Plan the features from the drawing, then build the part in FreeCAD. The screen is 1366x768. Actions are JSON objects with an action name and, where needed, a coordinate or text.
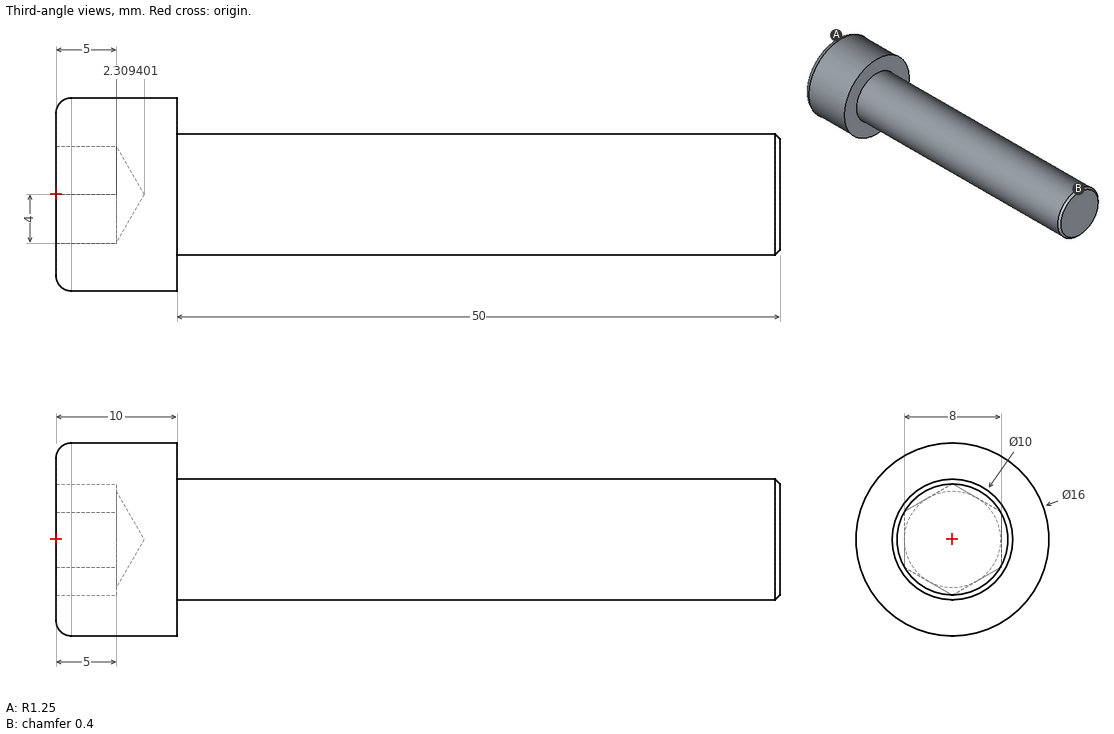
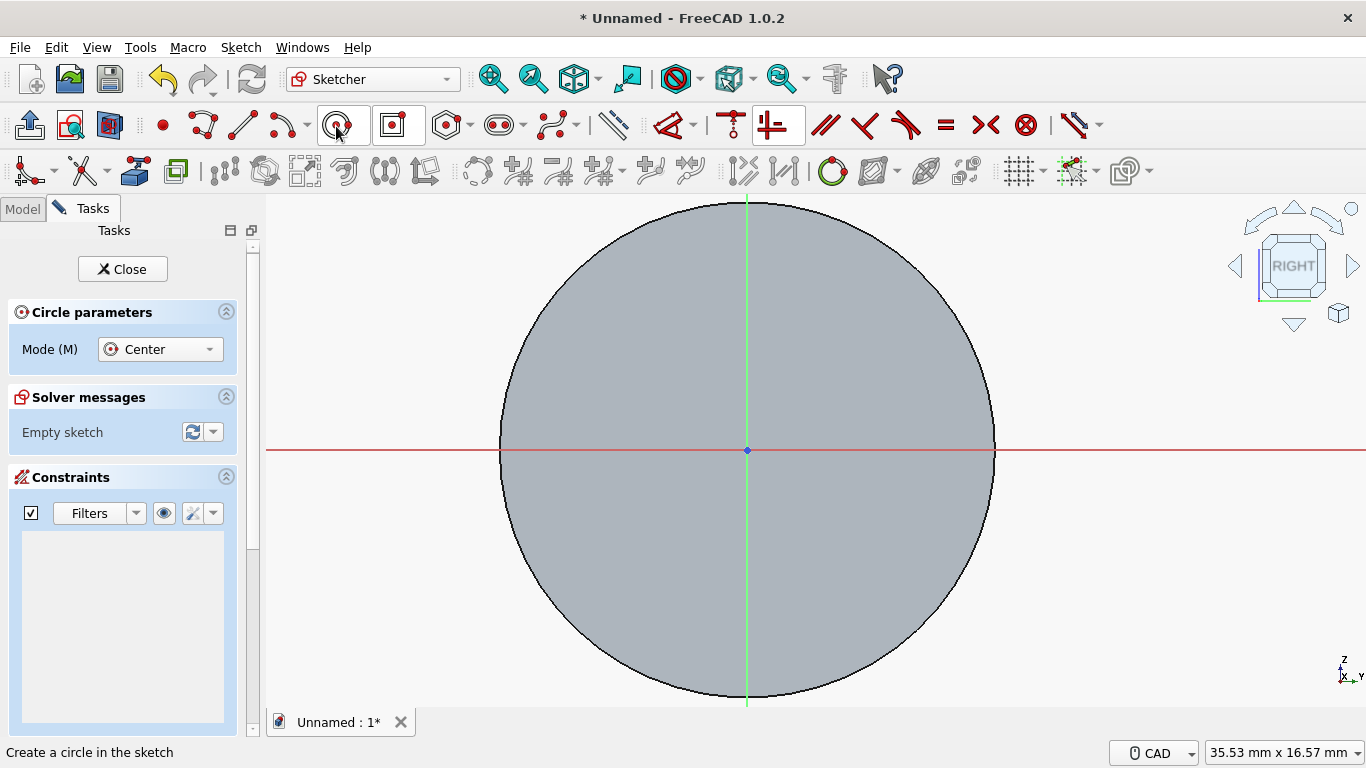
{"action": "left_click", "coordinate": [747, 450]}
{"action": "left_click", "coordinate": [857, 341]}
{"action": "key", "text": "Escape"}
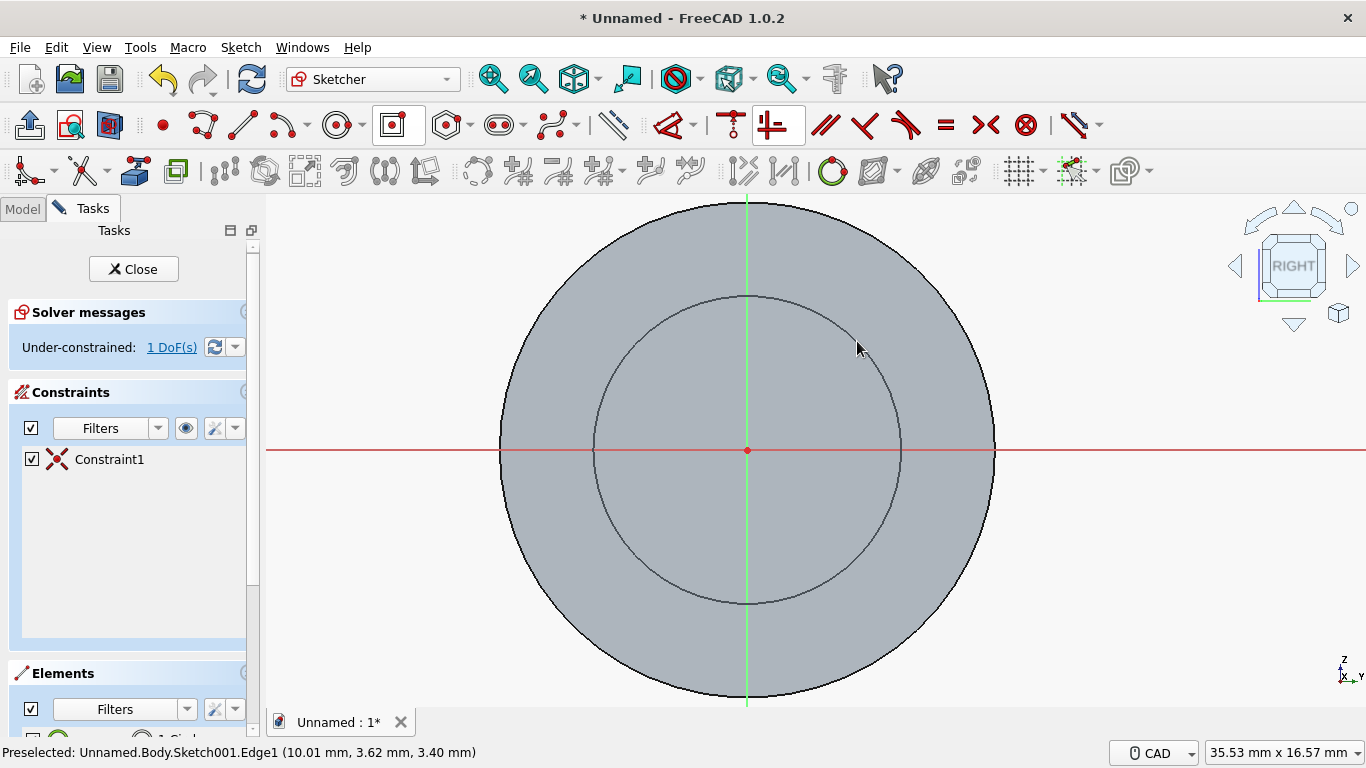
{"action": "left_click", "coordinate": [668, 126]}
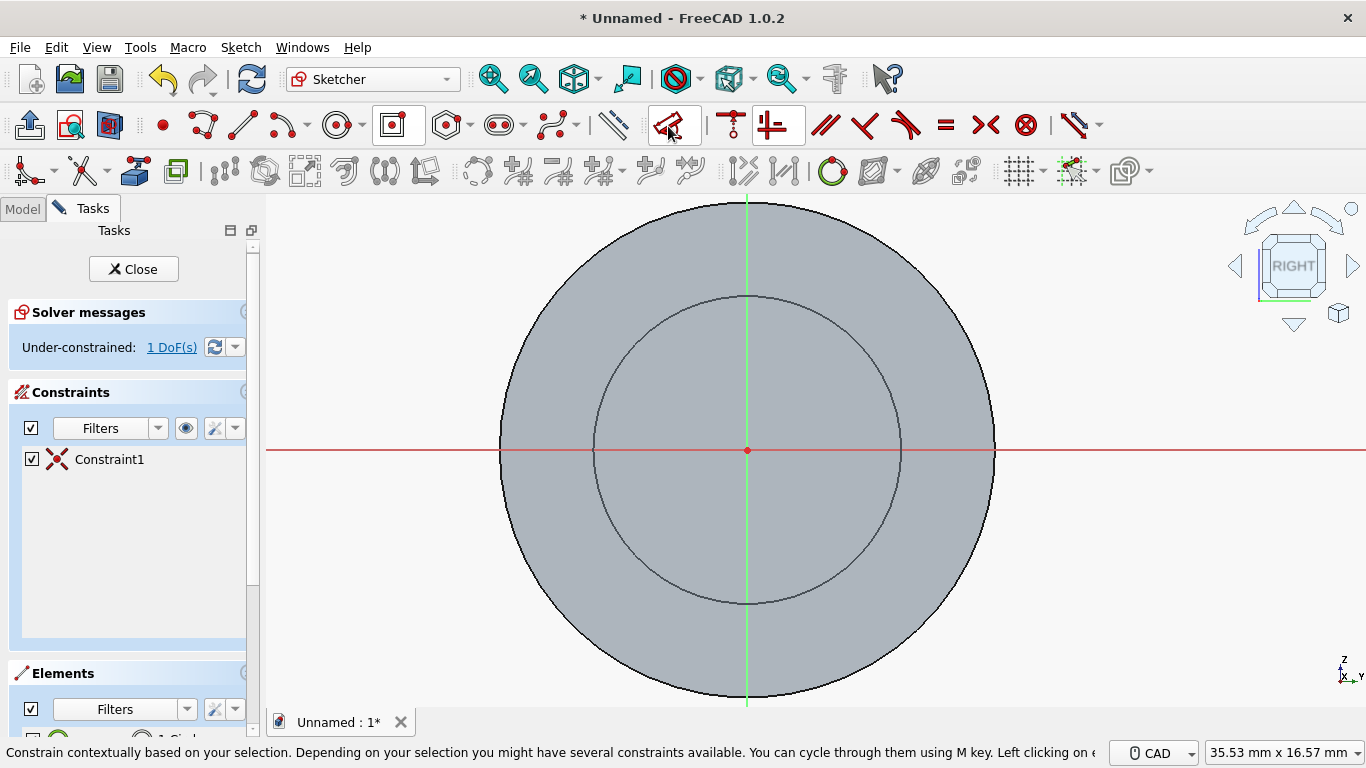
{"action": "left_click", "coordinate": [856, 341]}
{"action": "left_click", "coordinate": [879, 318]}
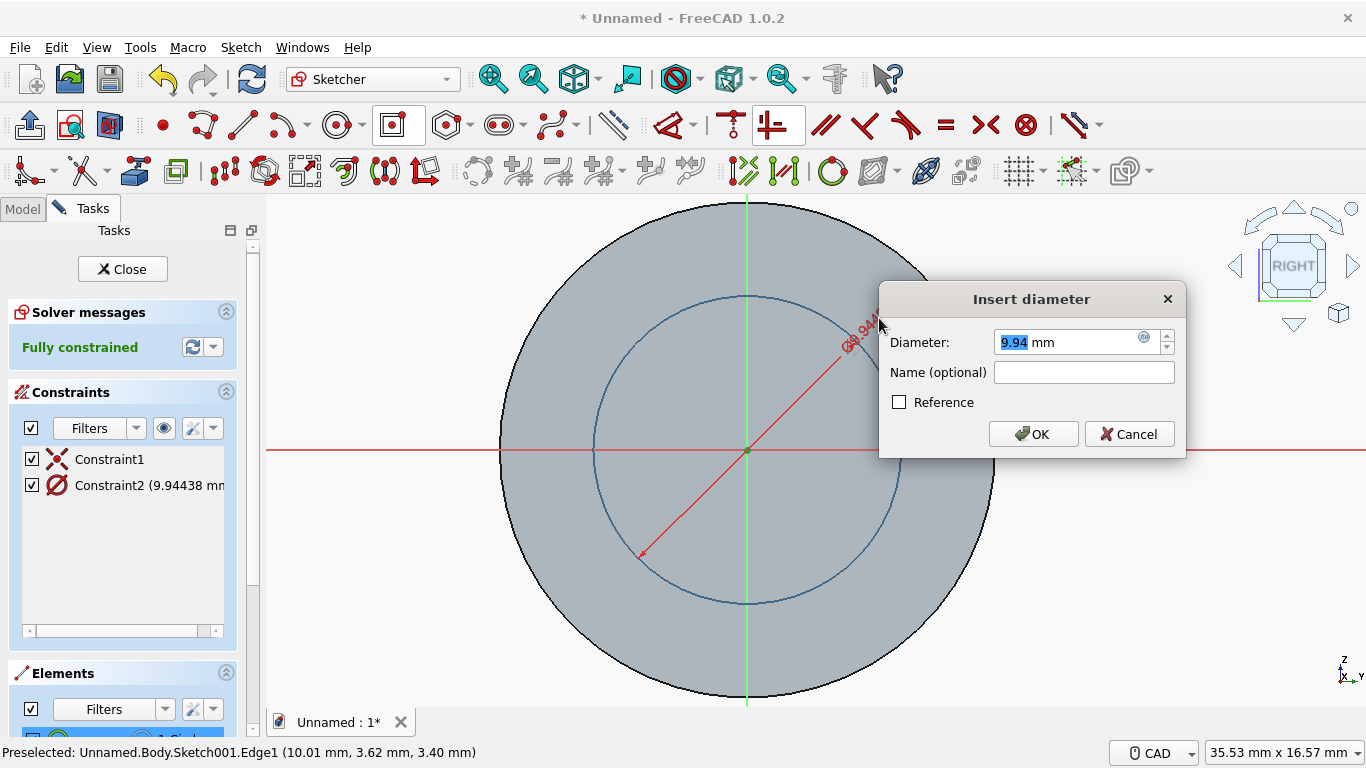
{"action": "type", "text": "10"}
{"action": "key", "text": "Return"}
{"action": "key", "text": "Escape"}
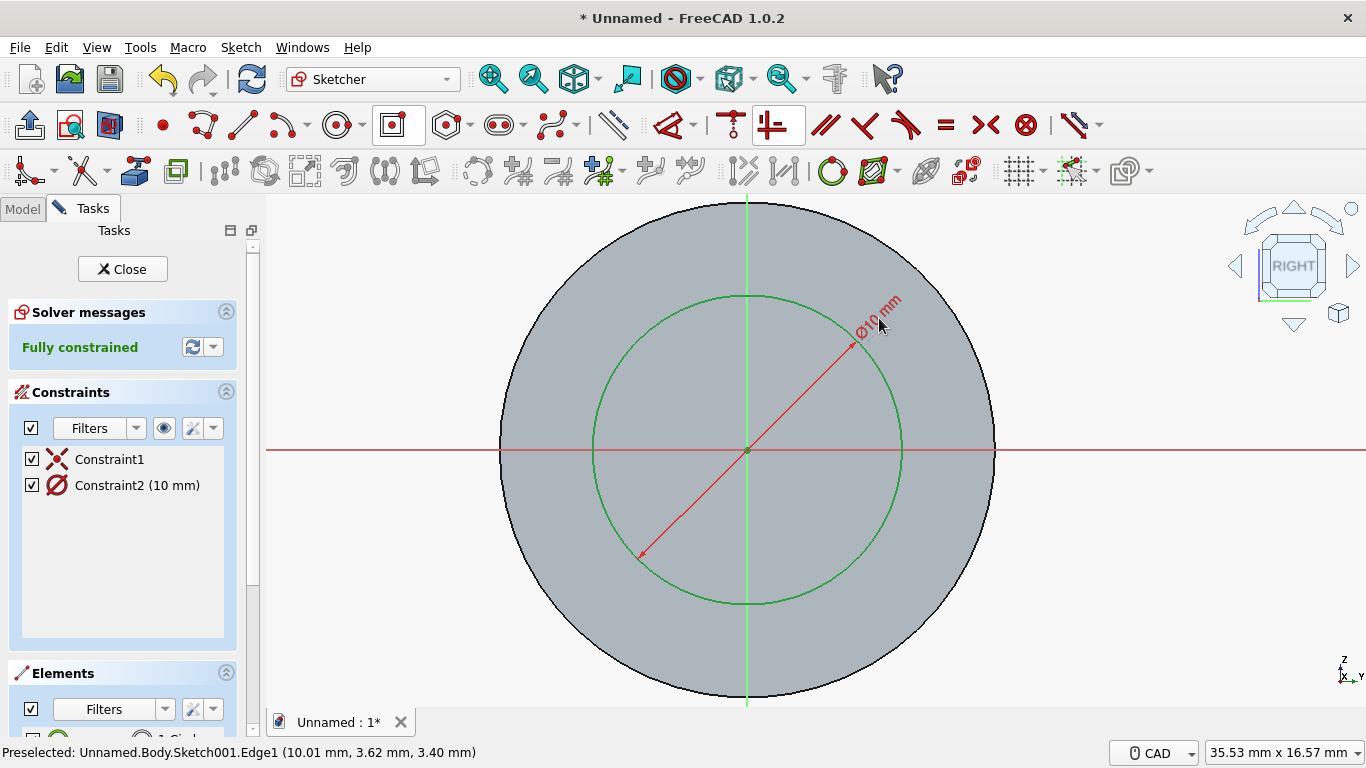
{"action": "left_click", "coordinate": [123, 269]}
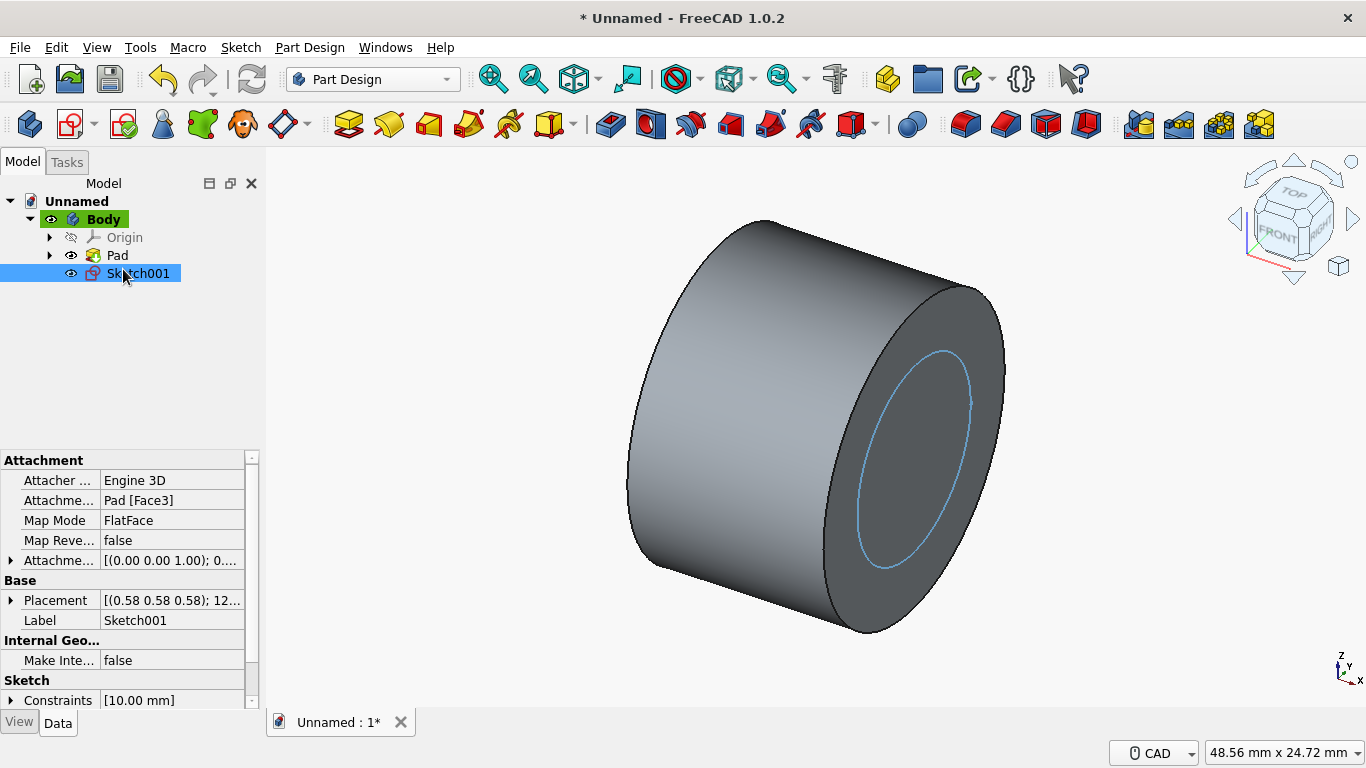
{"action": "left_click", "coordinate": [350, 124]}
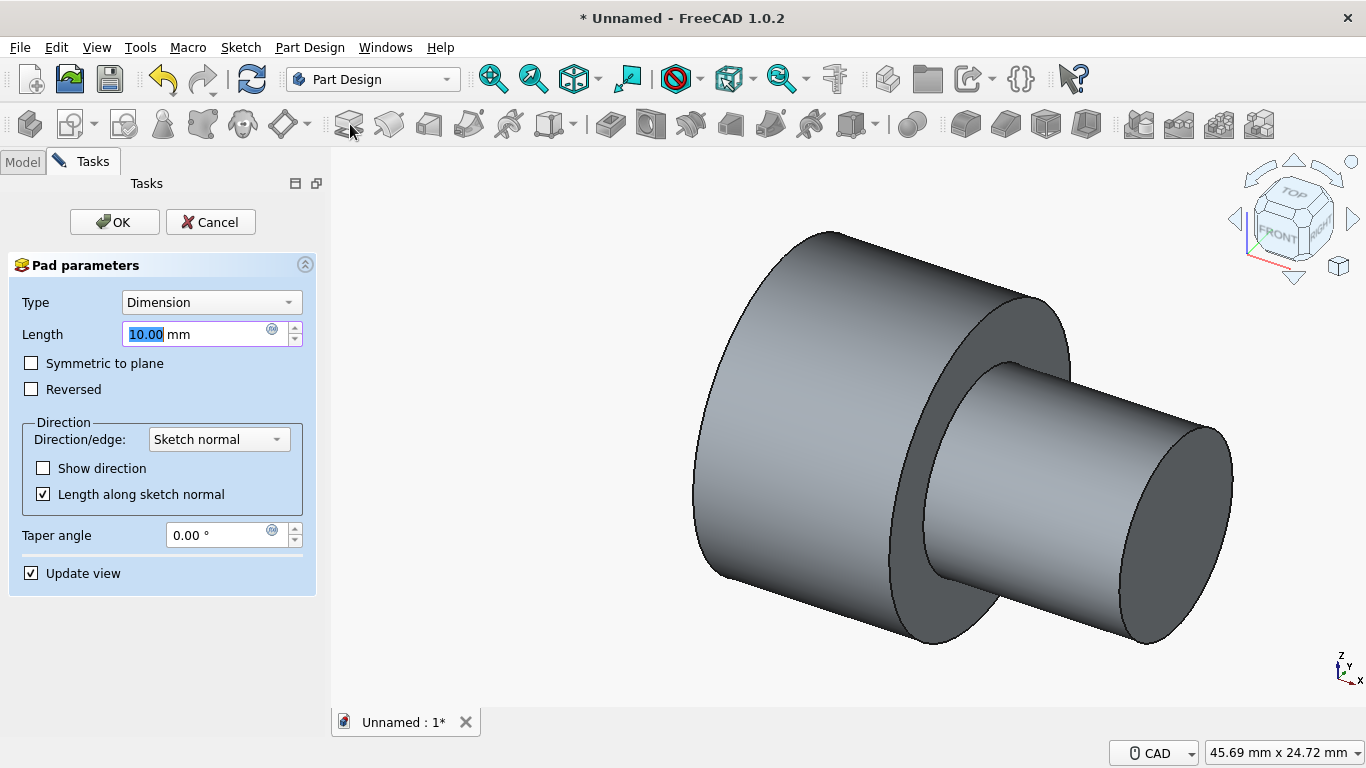
{"action": "type", "text": "50"}
{"action": "key", "text": "Tab"}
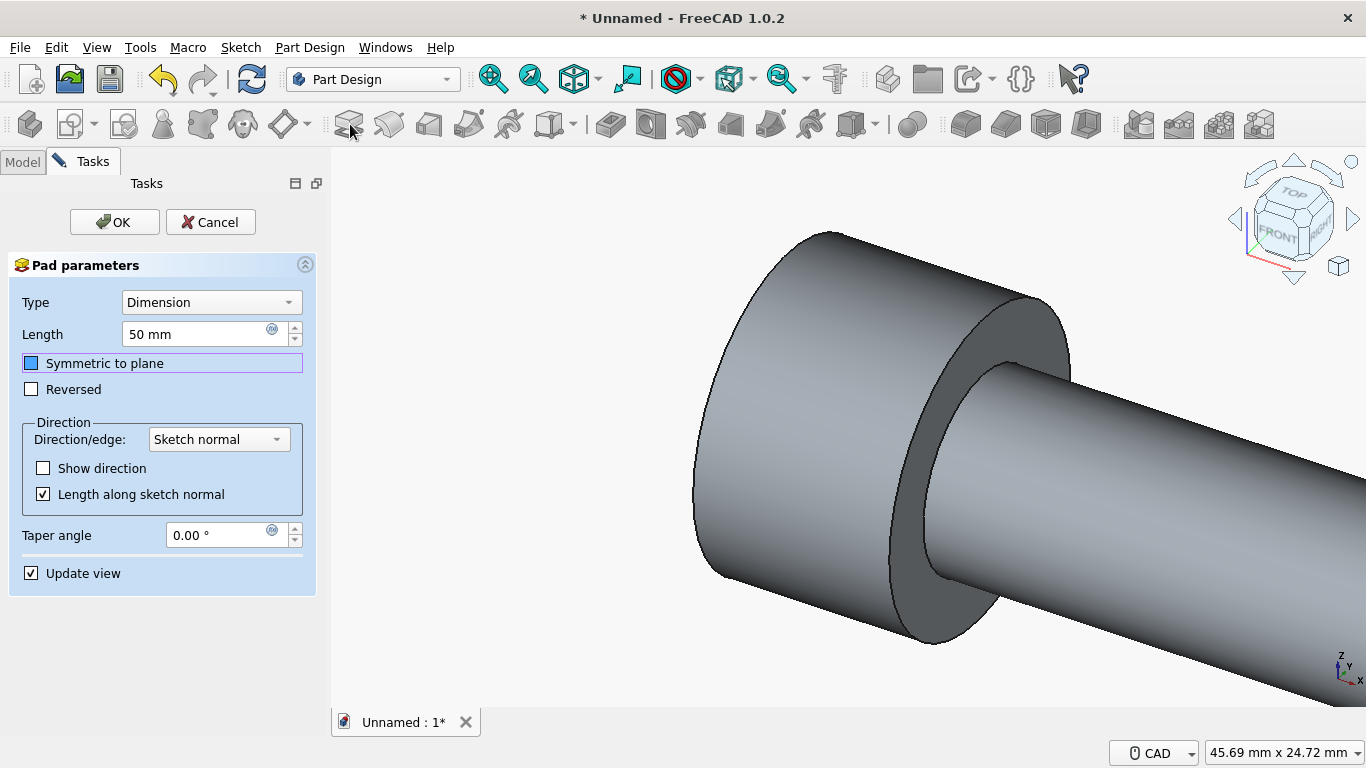
{"action": "left_click", "coordinate": [115, 222]}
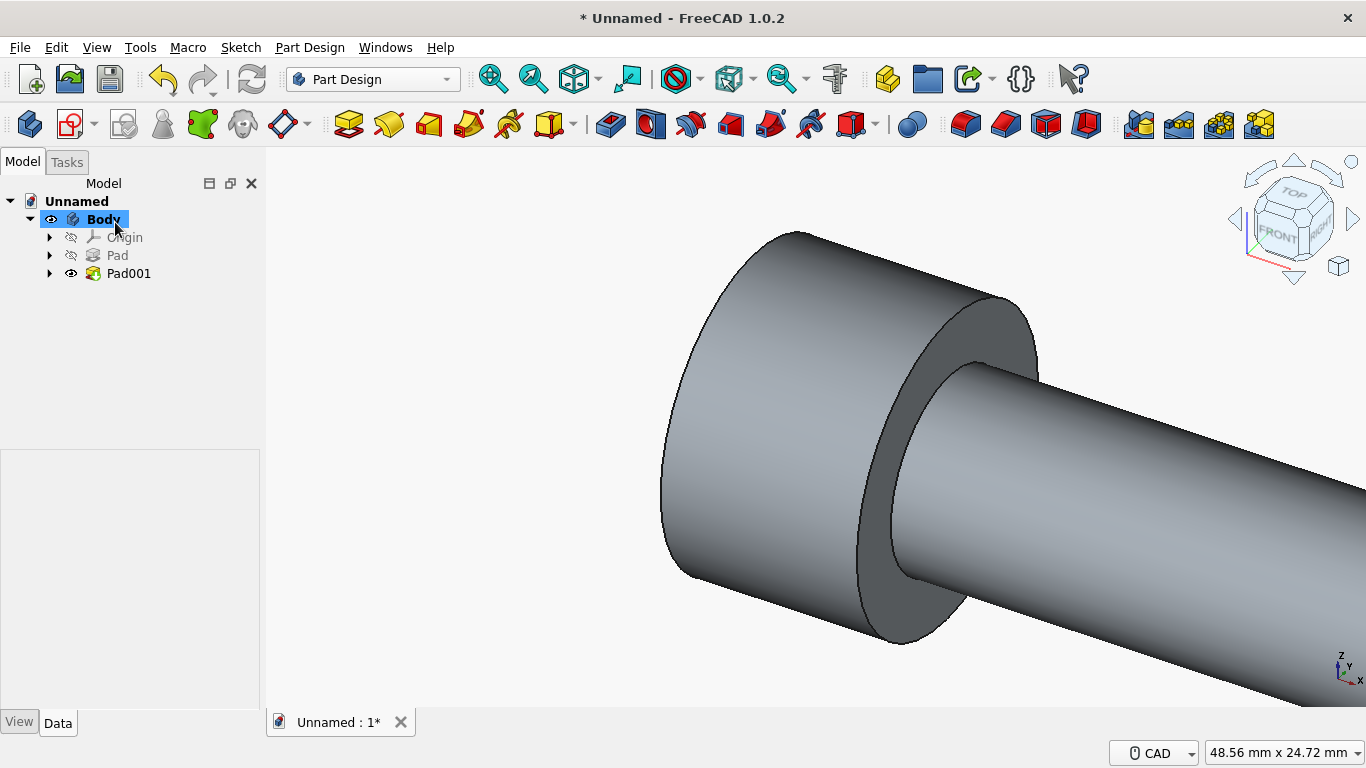
{"action": "left_click", "coordinate": [494, 80]}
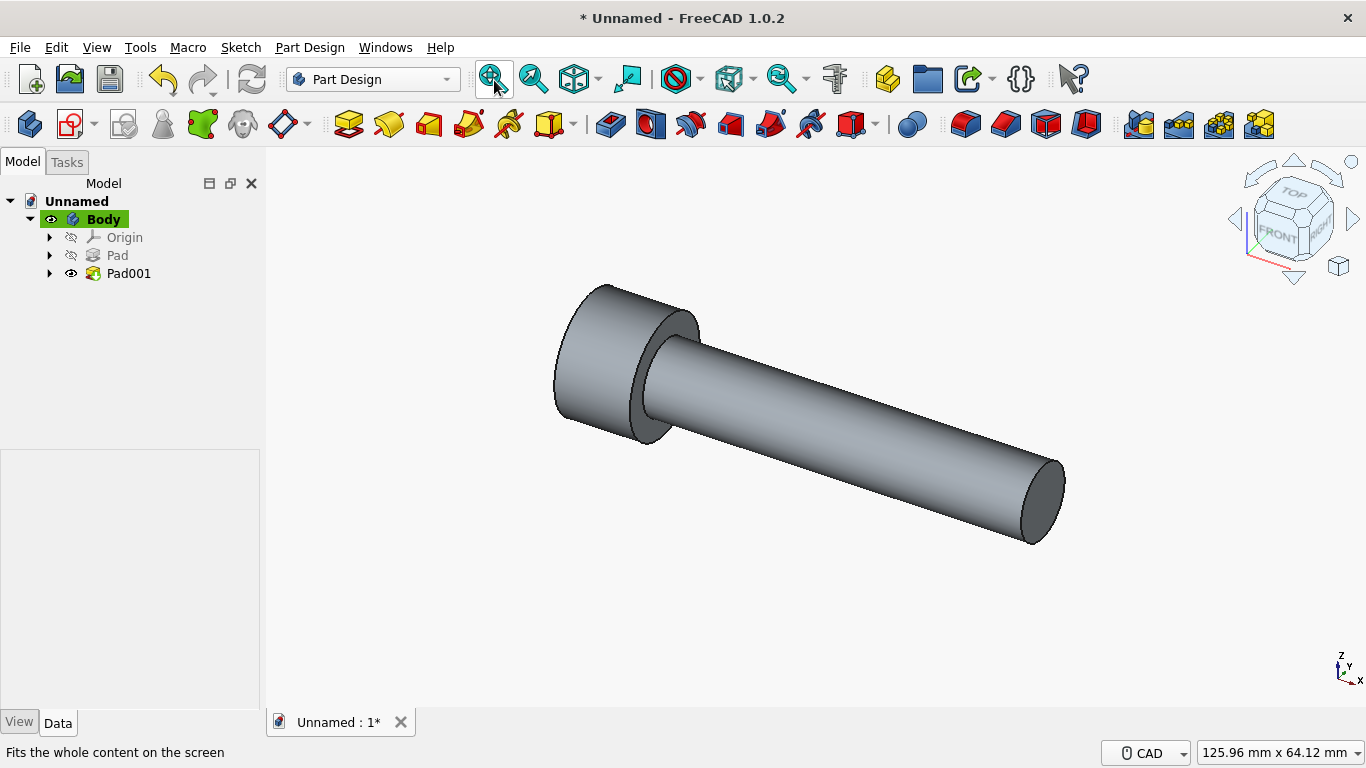
{"action": "left_click", "coordinate": [70, 124]}